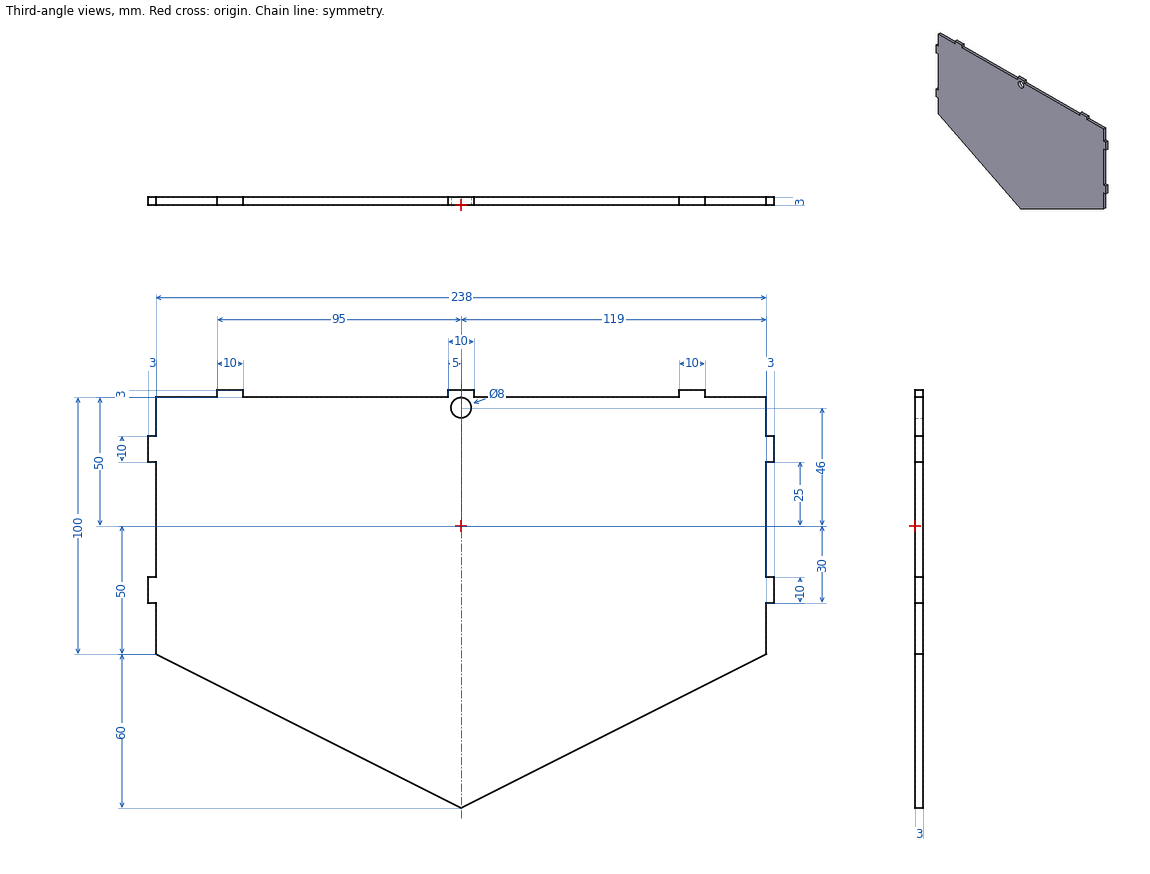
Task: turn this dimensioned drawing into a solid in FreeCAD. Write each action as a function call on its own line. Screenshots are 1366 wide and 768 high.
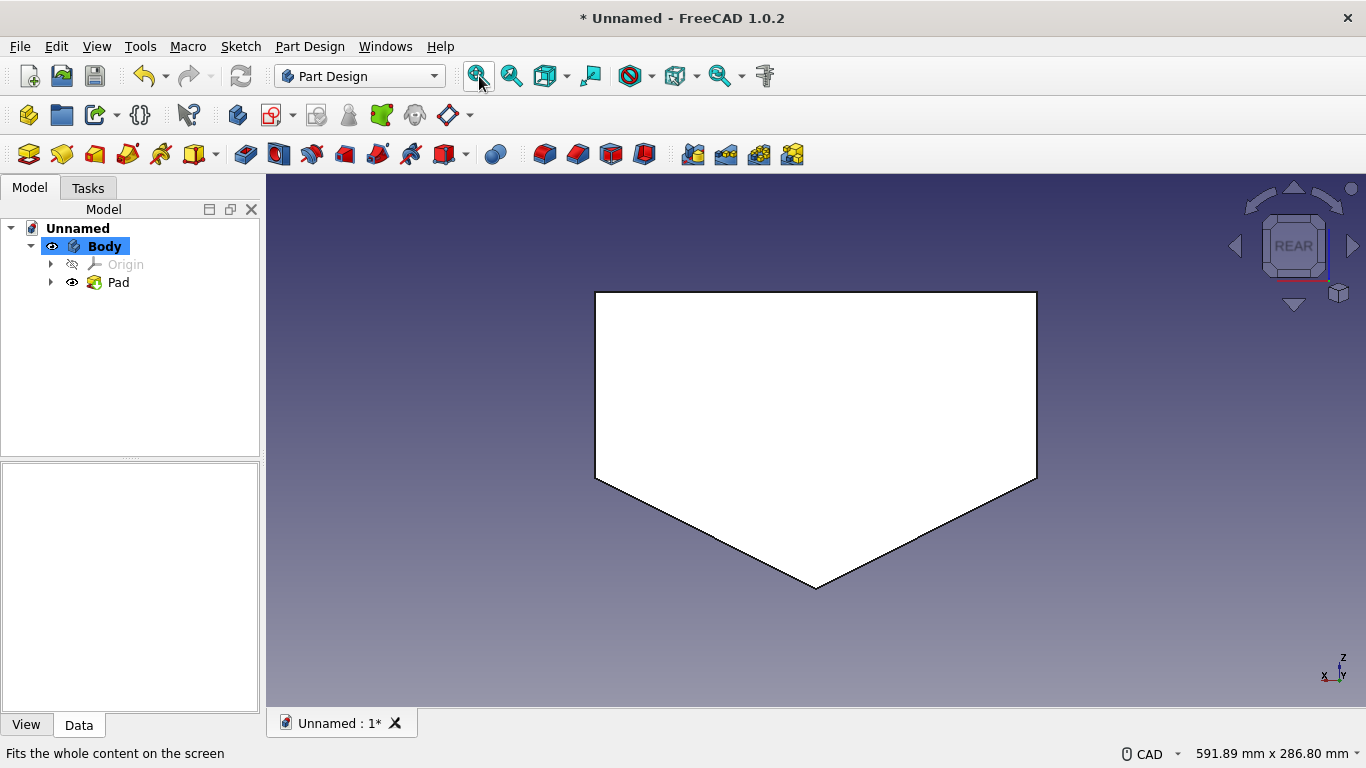
click(816, 439)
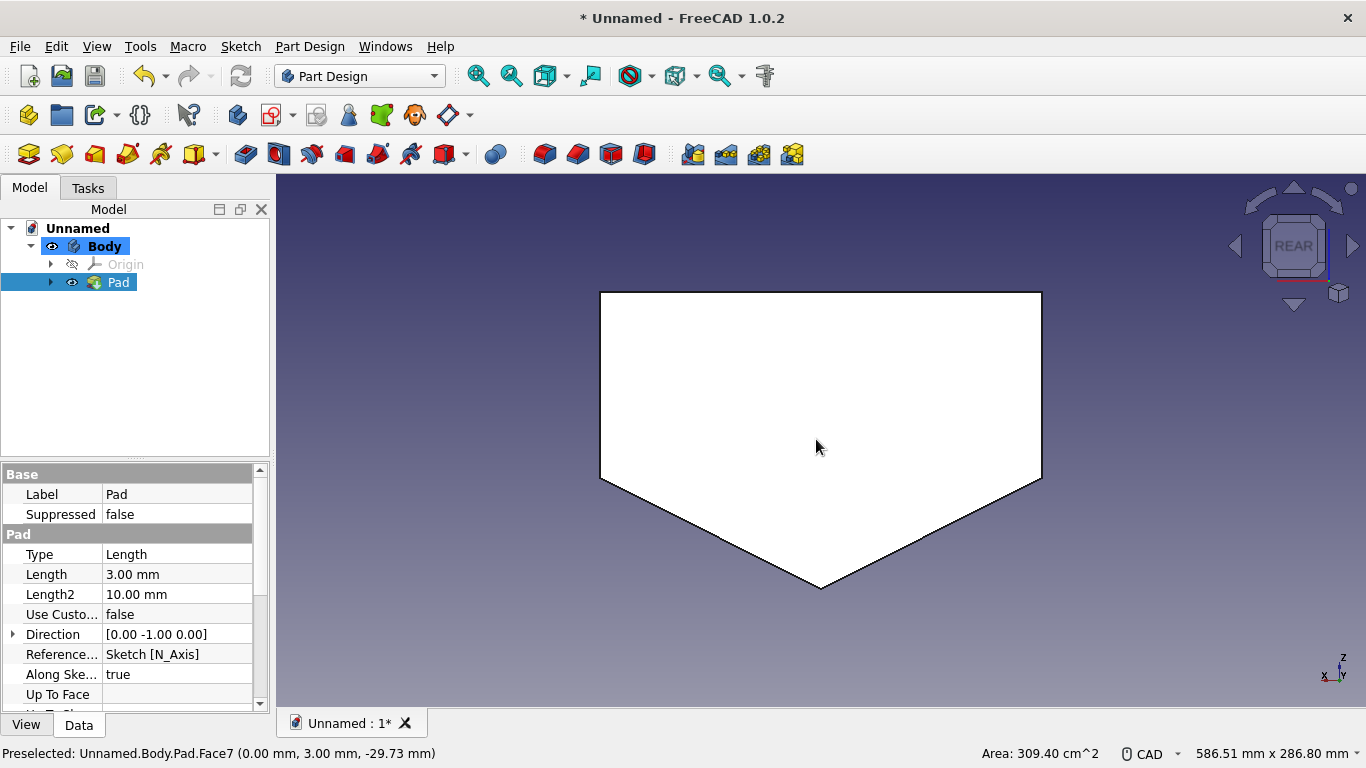
click(270, 116)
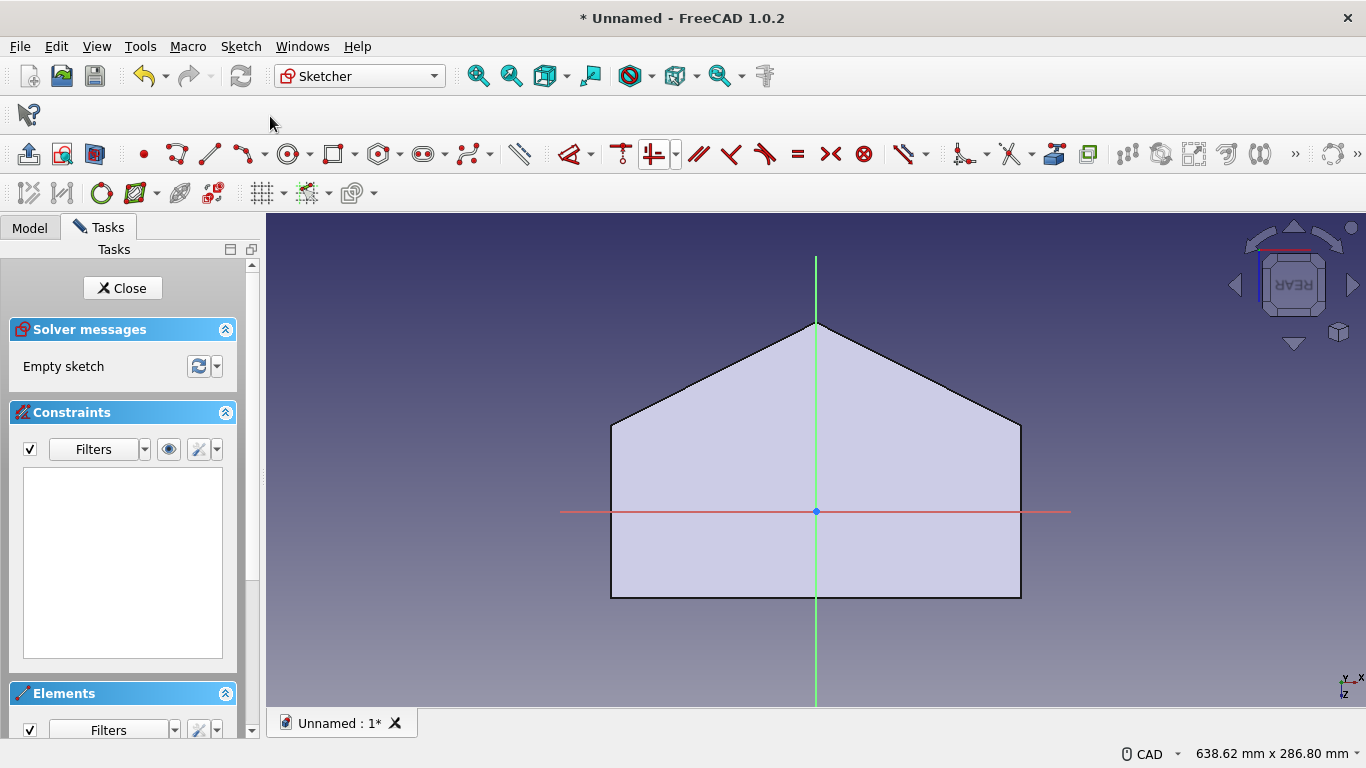
scroll(955, 677, up, 2)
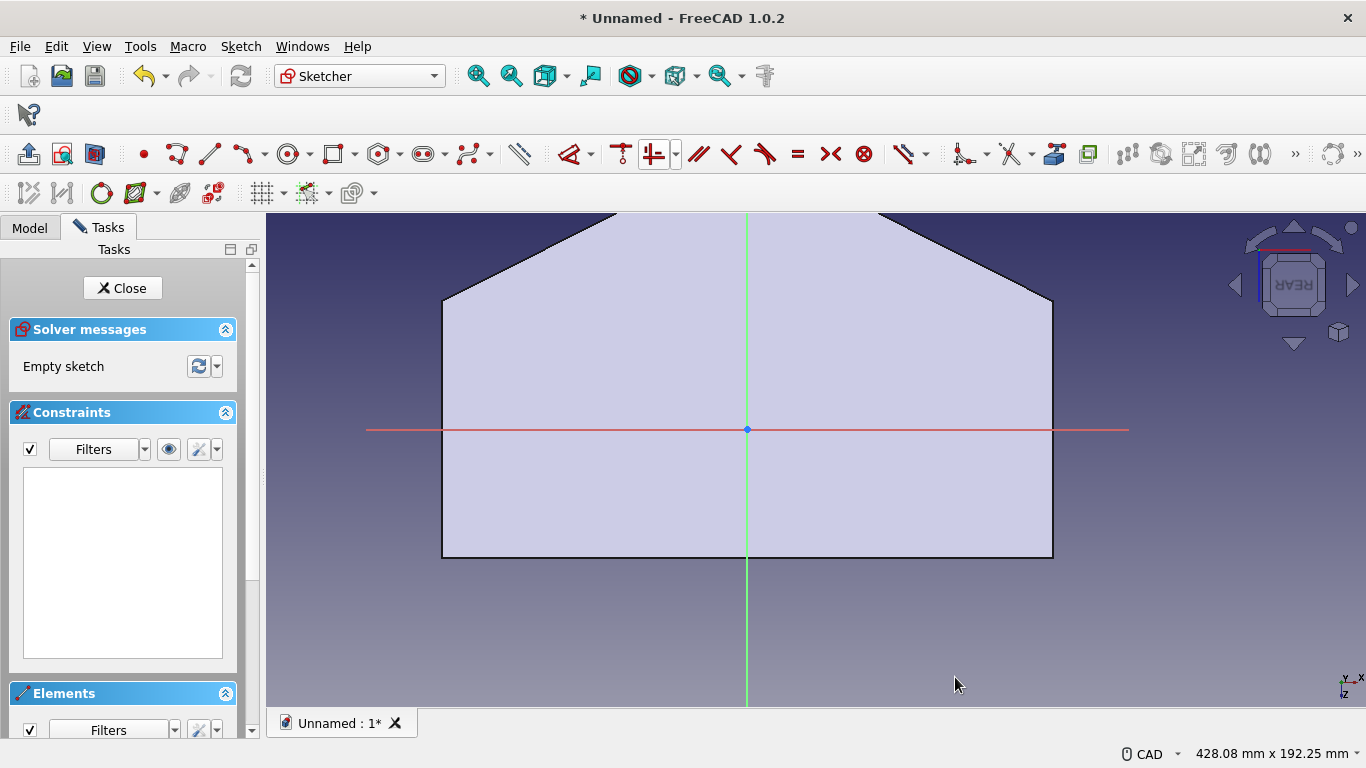
click(332, 154)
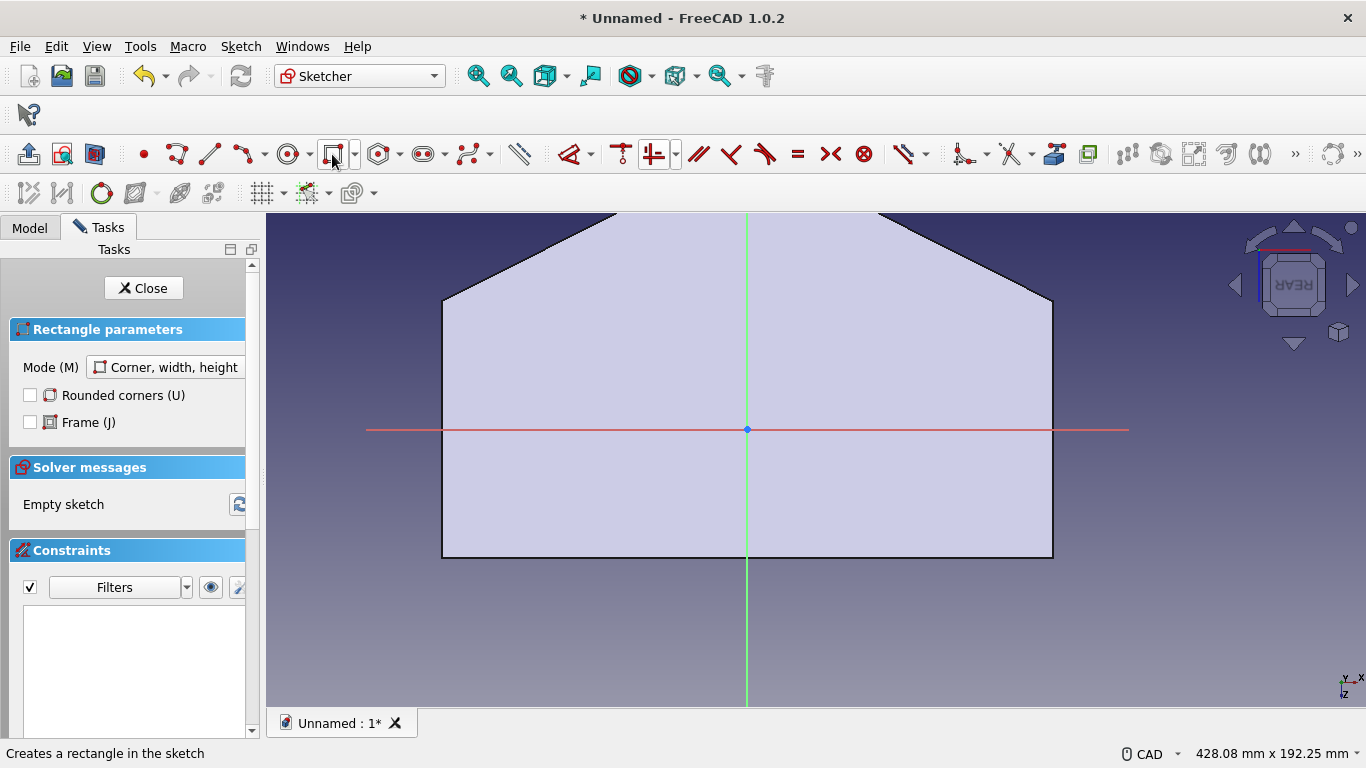
scroll(1053, 353, up, 4)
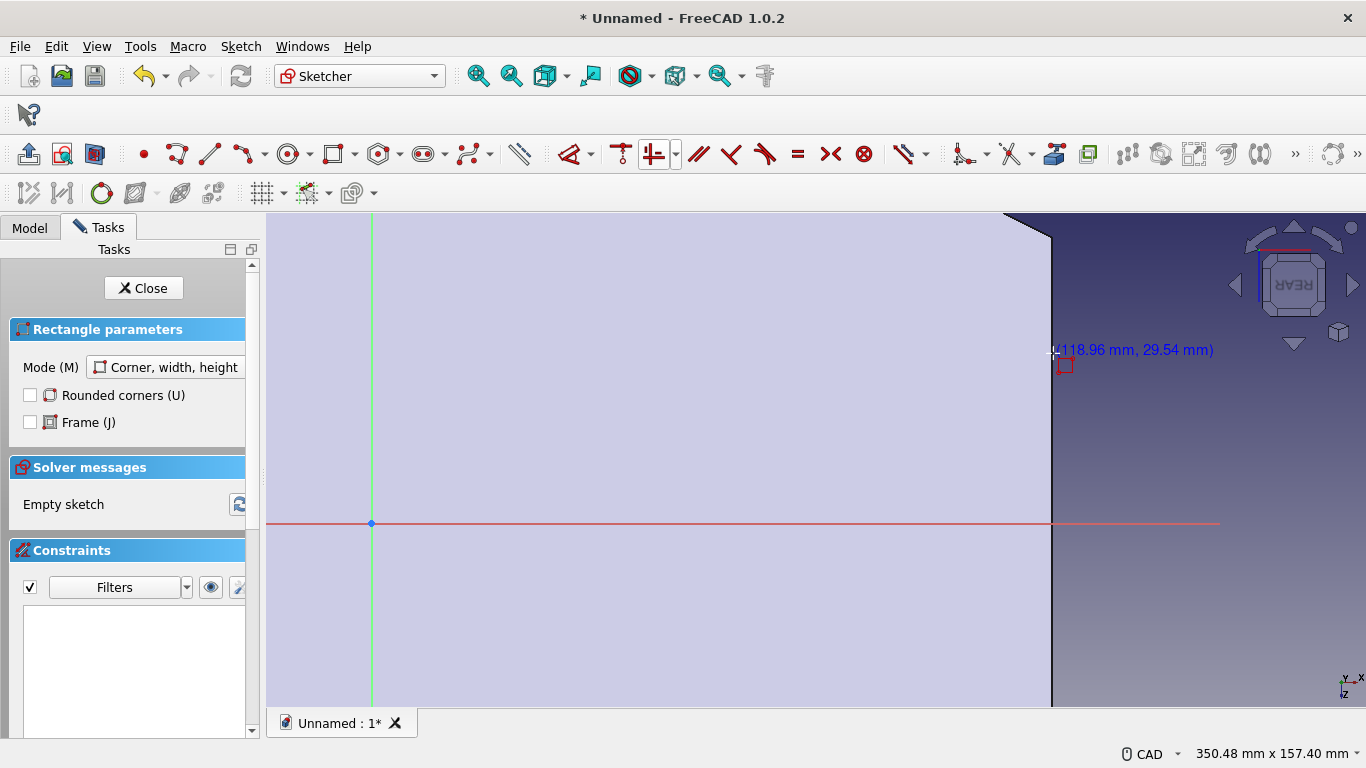
click(1052, 352)
move(1070, 409)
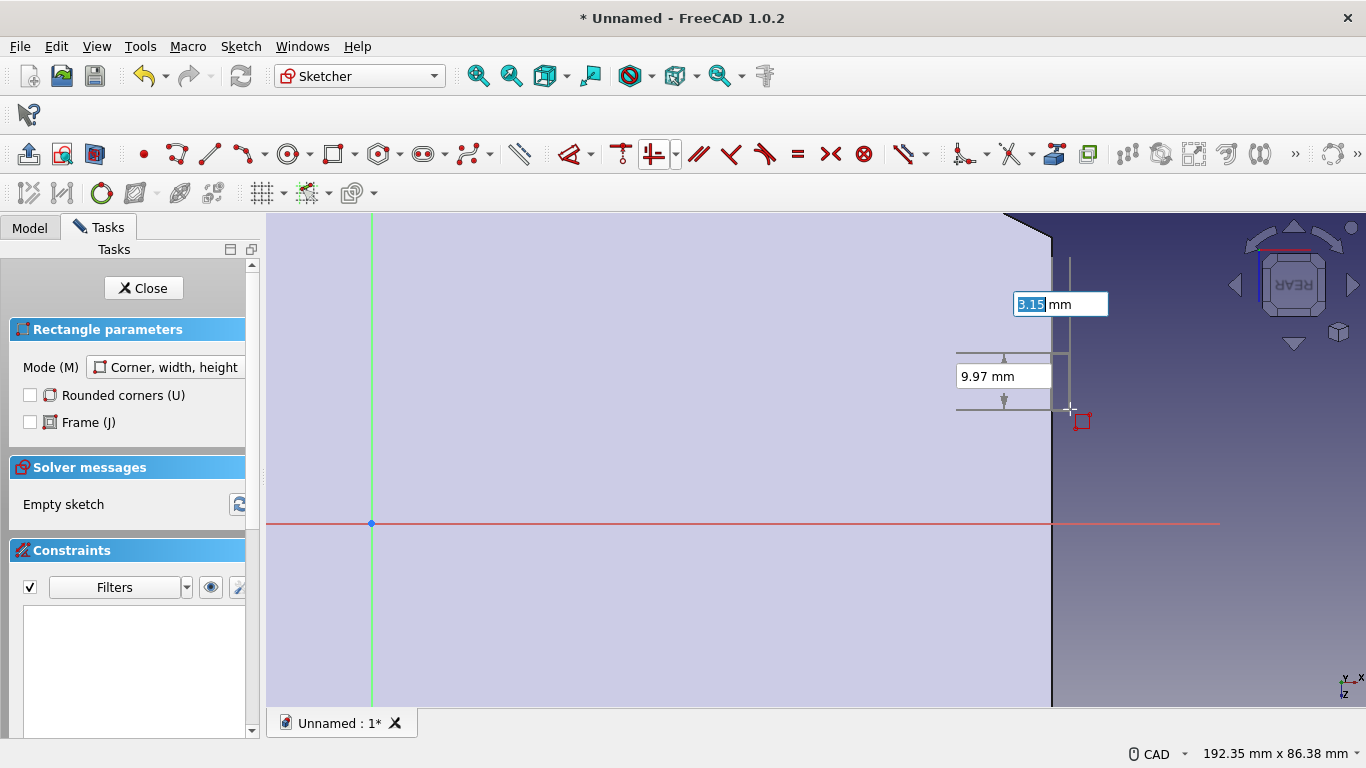
text(3)
key(Tab)
text(10)
key(Return)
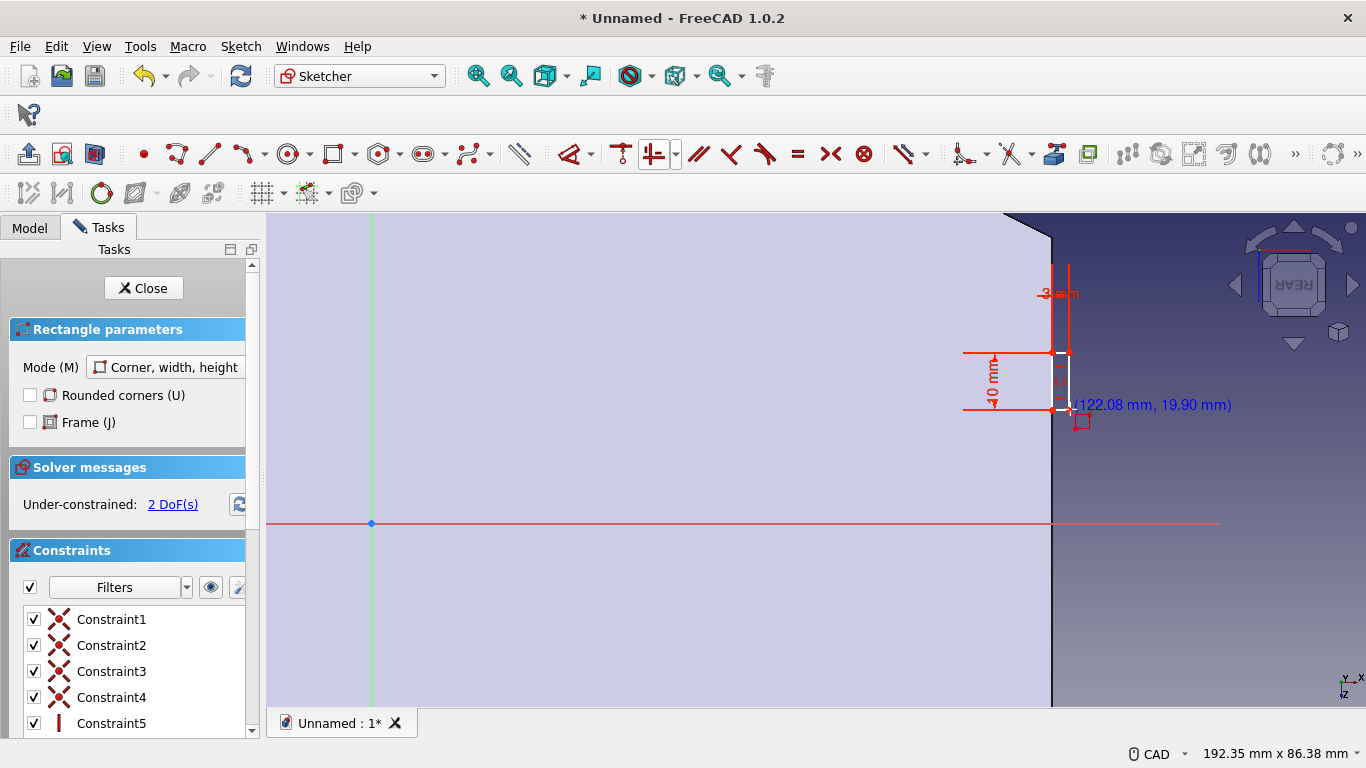
click(1052, 667)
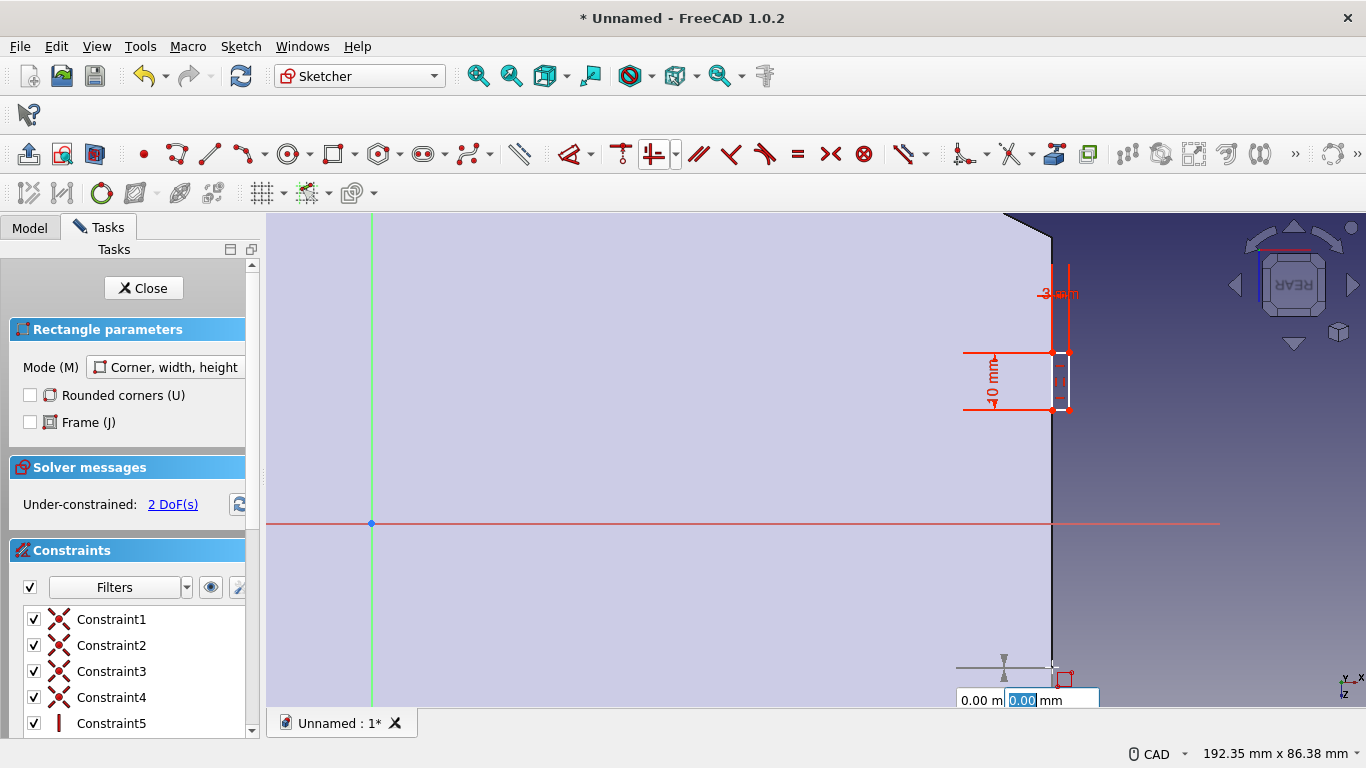
scroll(1054, 354, down, 4)